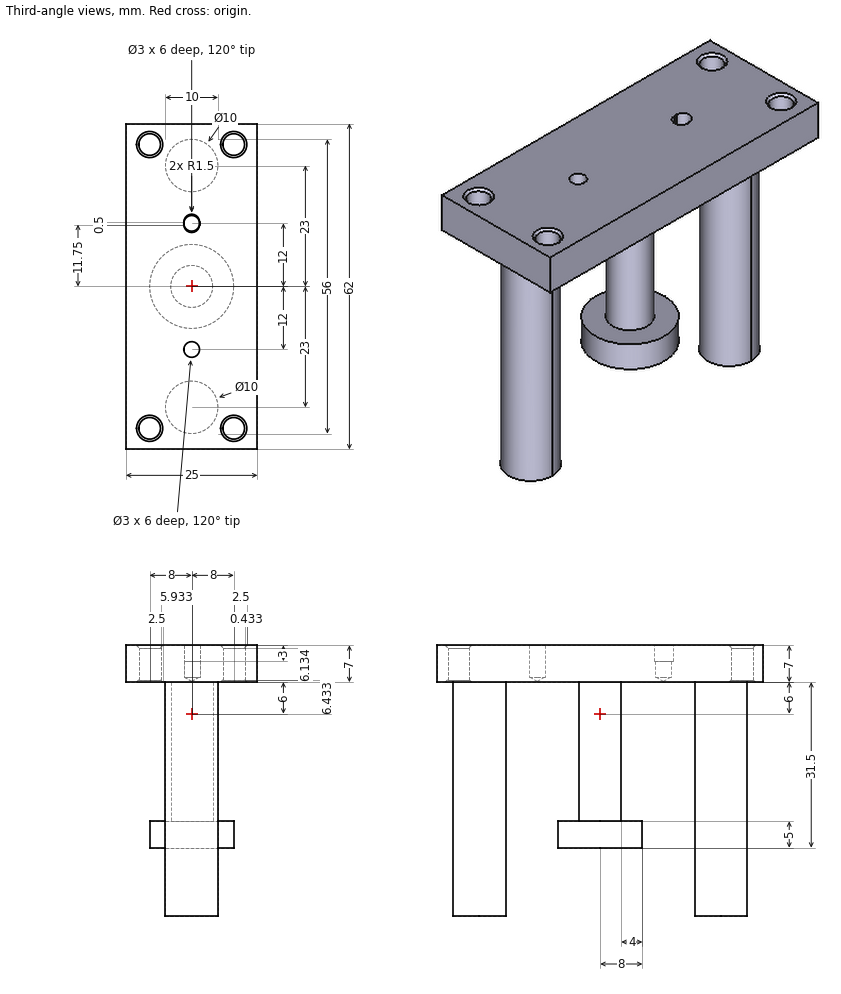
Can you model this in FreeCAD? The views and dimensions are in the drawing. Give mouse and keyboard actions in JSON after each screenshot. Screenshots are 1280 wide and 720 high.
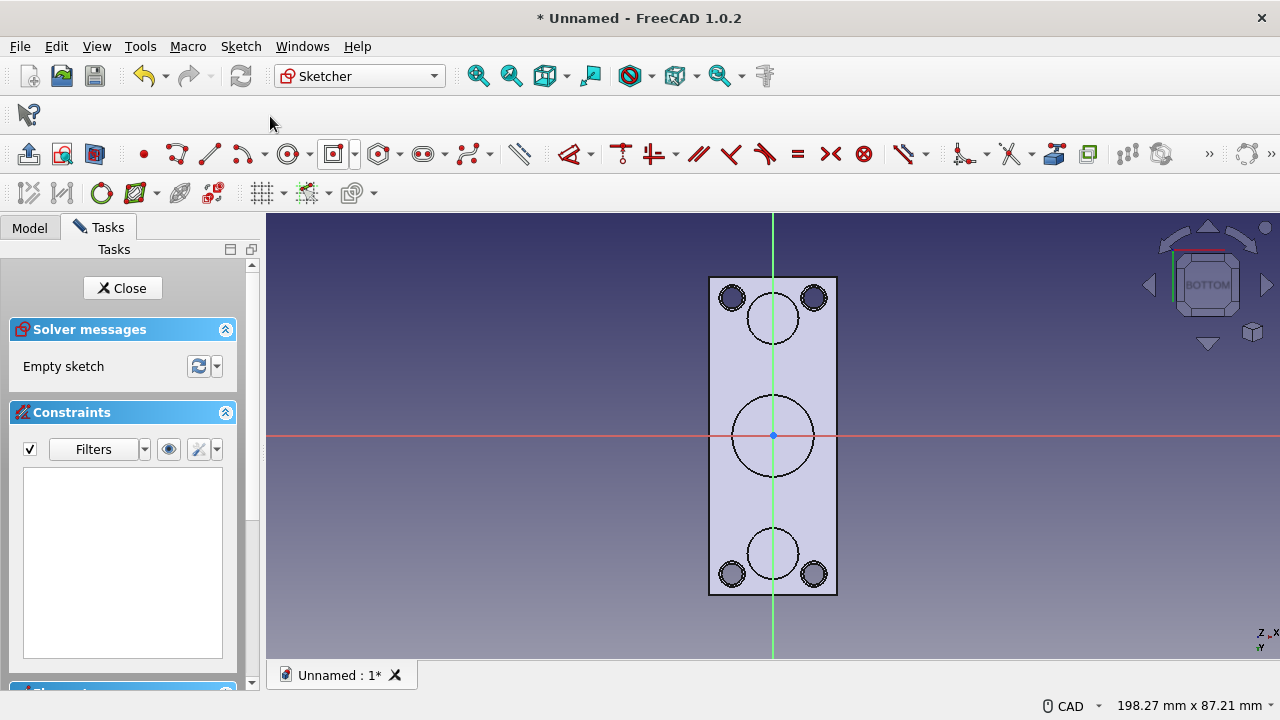
{"action": "left_click", "coordinate": [332, 154]}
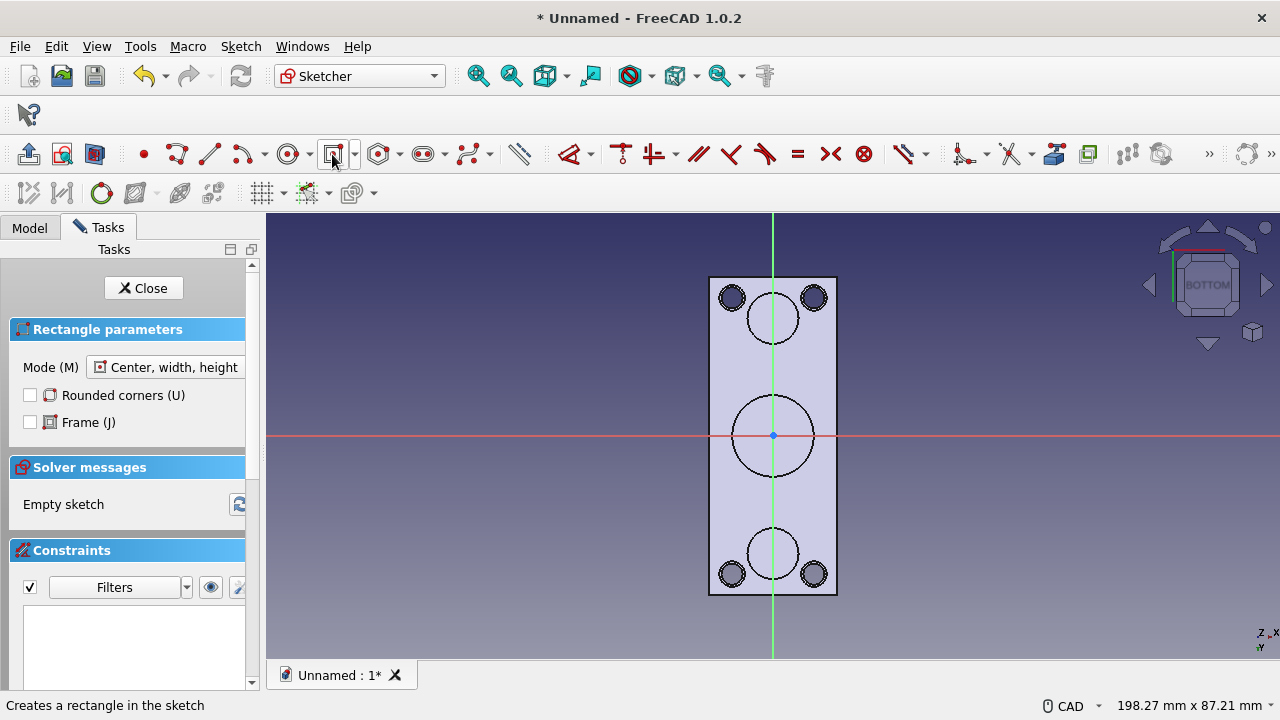
{"action": "left_click", "coordinate": [773, 436]}
{"action": "left_click", "coordinate": [799, 293]}
{"action": "key", "text": "Escape"}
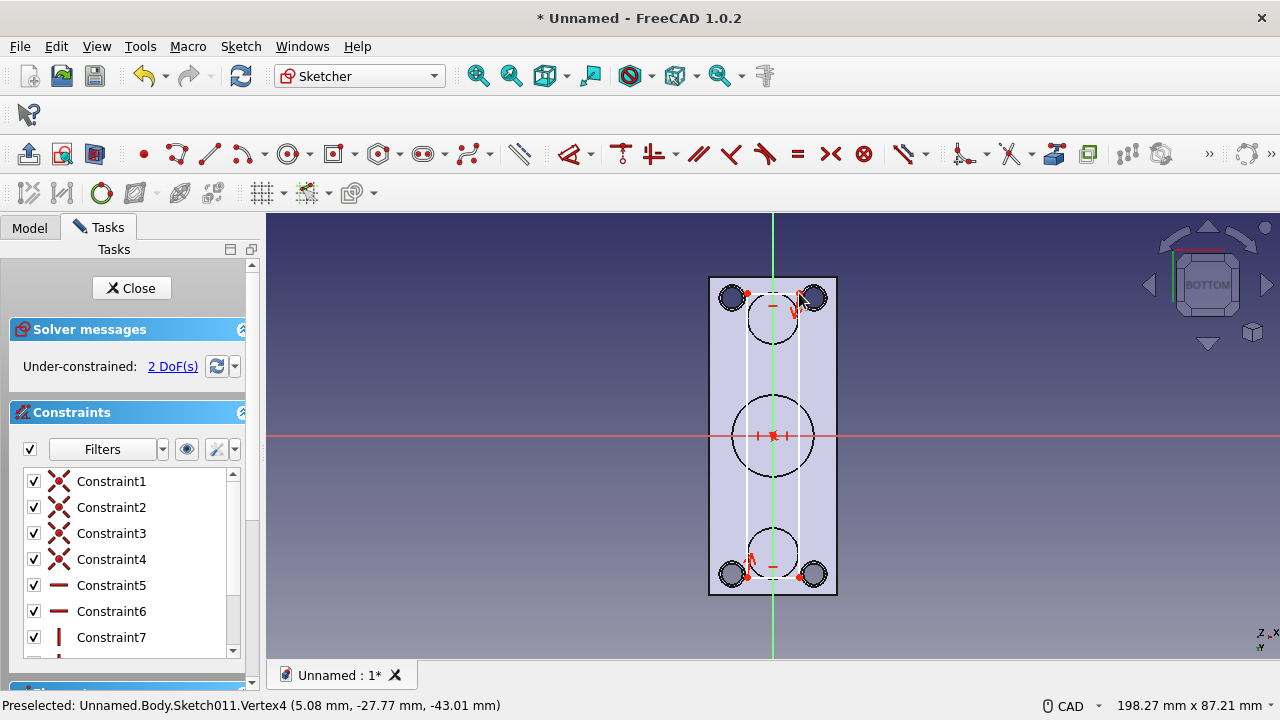
{"action": "left_click", "coordinate": [568, 154]}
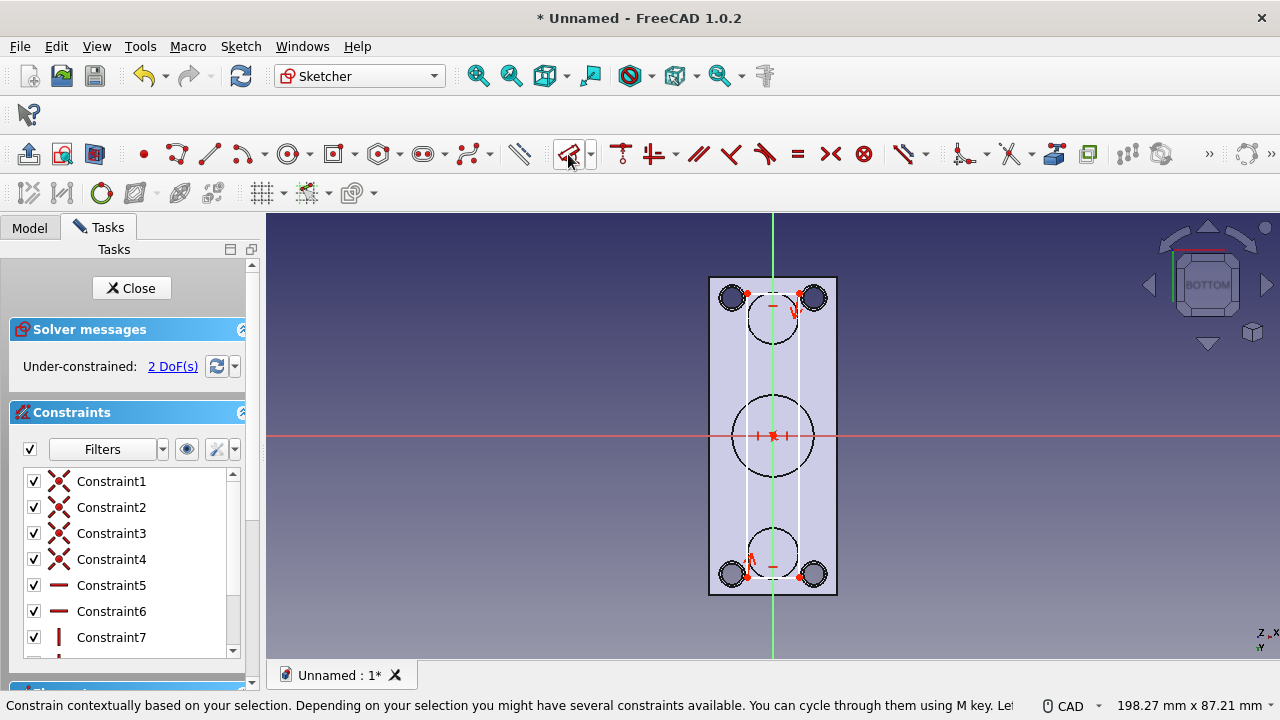
{"action": "scroll", "coordinate": [763, 578], "scroll_direction": "up", "scroll_amount": 2}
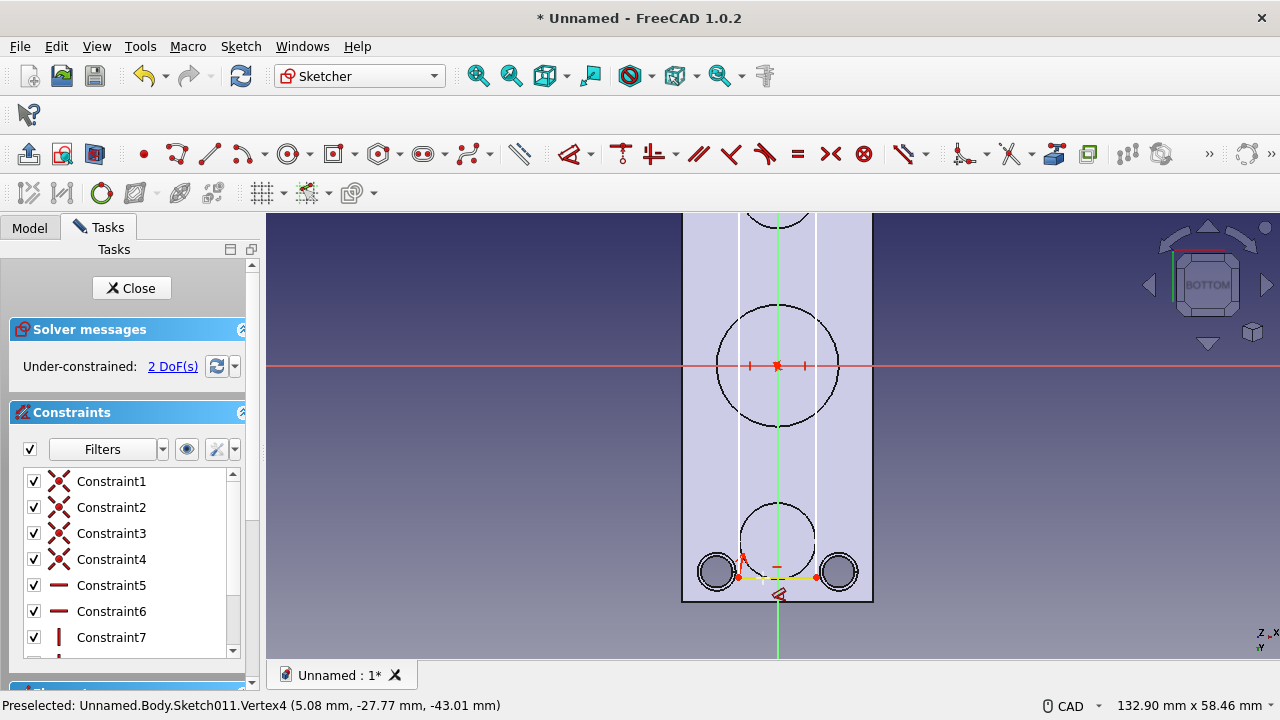
{"action": "left_click", "coordinate": [762, 578]}
{"action": "left_click", "coordinate": [760, 612]}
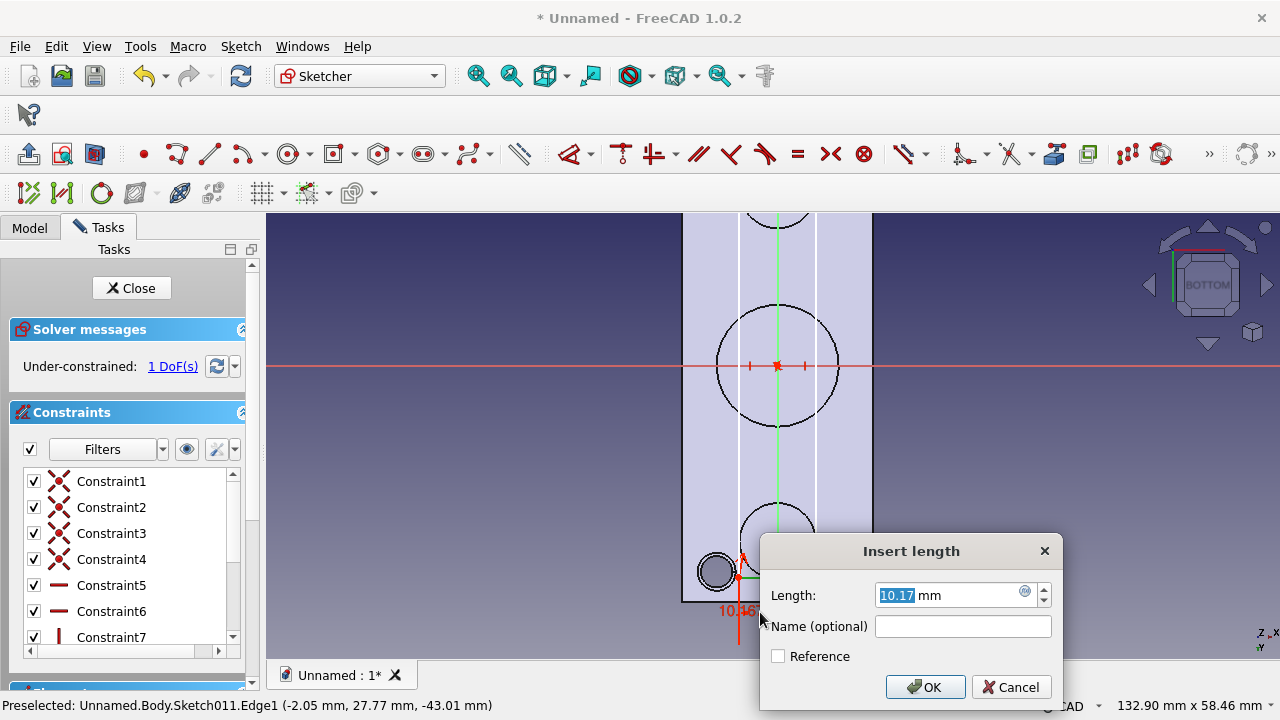
{"action": "type", "text": "10"}
{"action": "key", "text": "Return"}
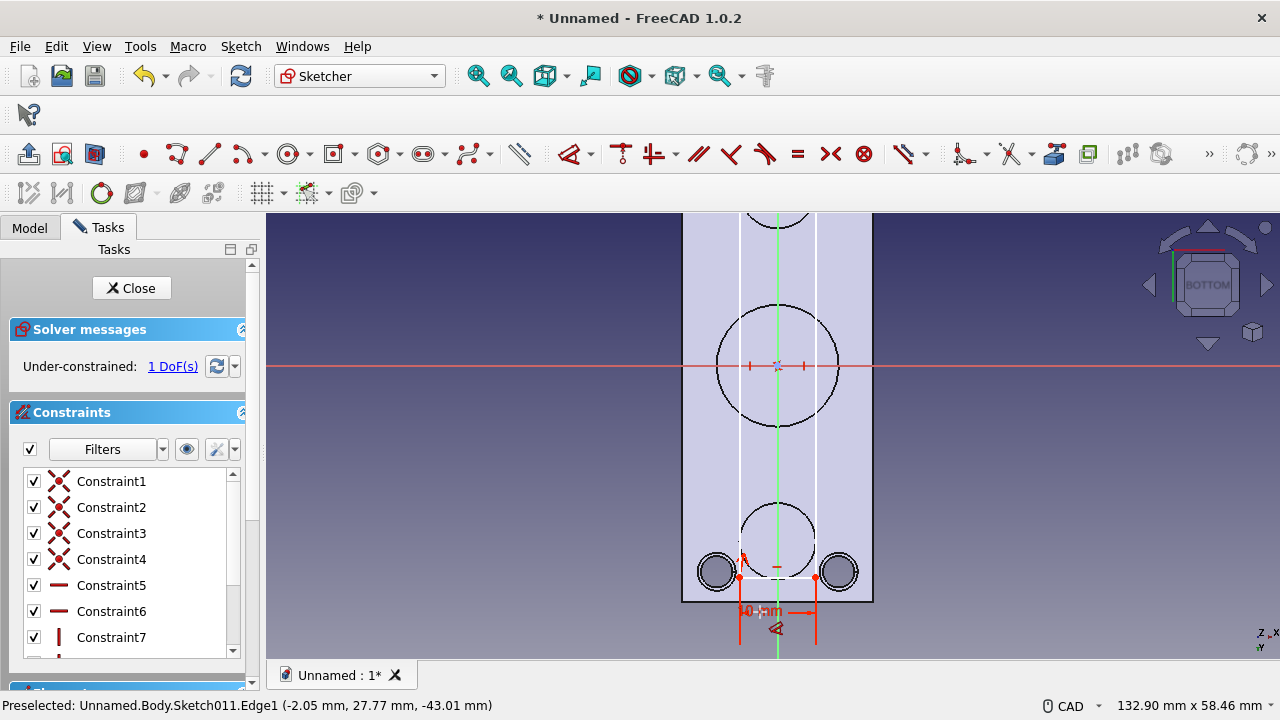
{"action": "left_click", "coordinate": [816, 450]}
{"action": "left_click", "coordinate": [850, 409]}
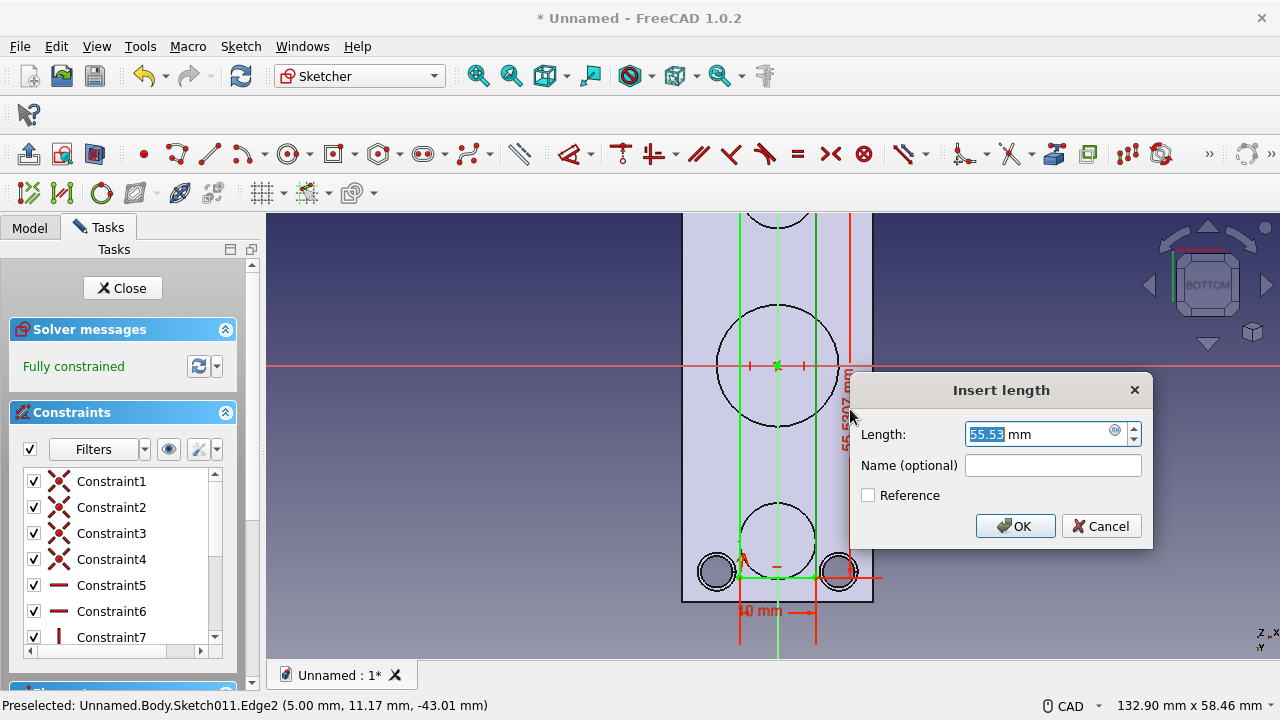
{"action": "type", "text": "56"}
{"action": "key", "text": "Return"}
{"action": "key", "text": "Escape"}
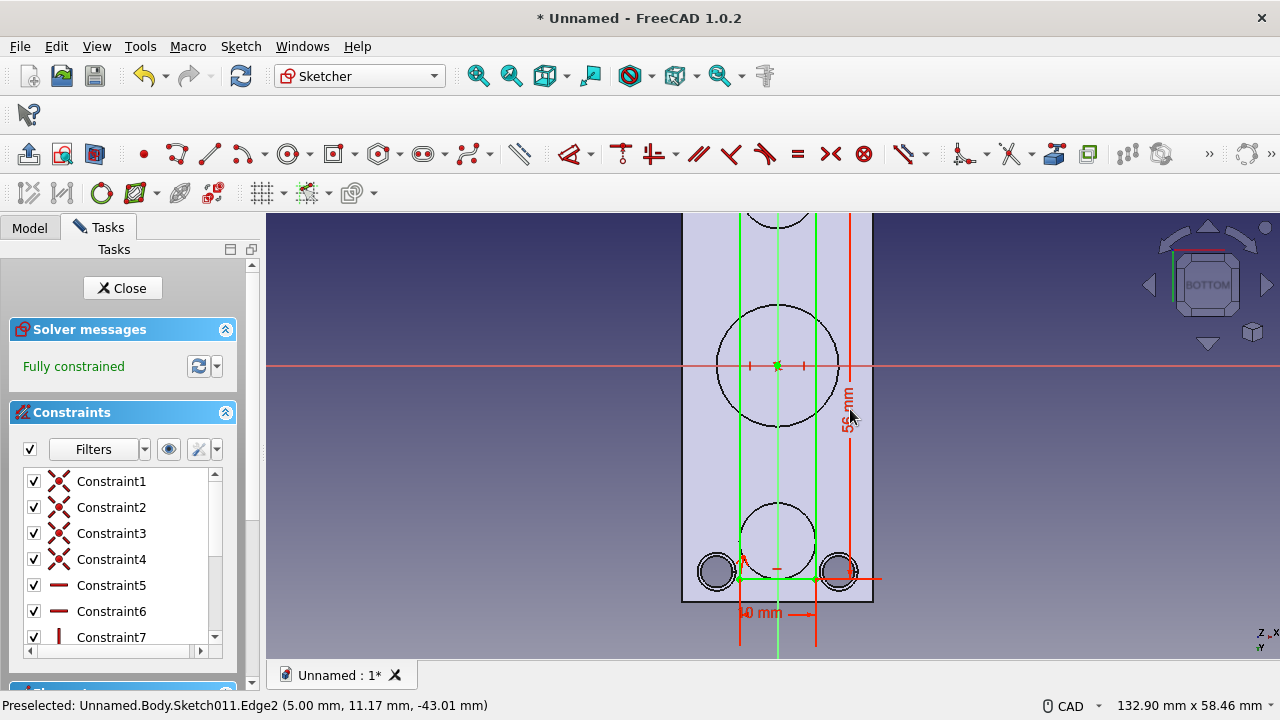
{"action": "left_click", "coordinate": [123, 288]}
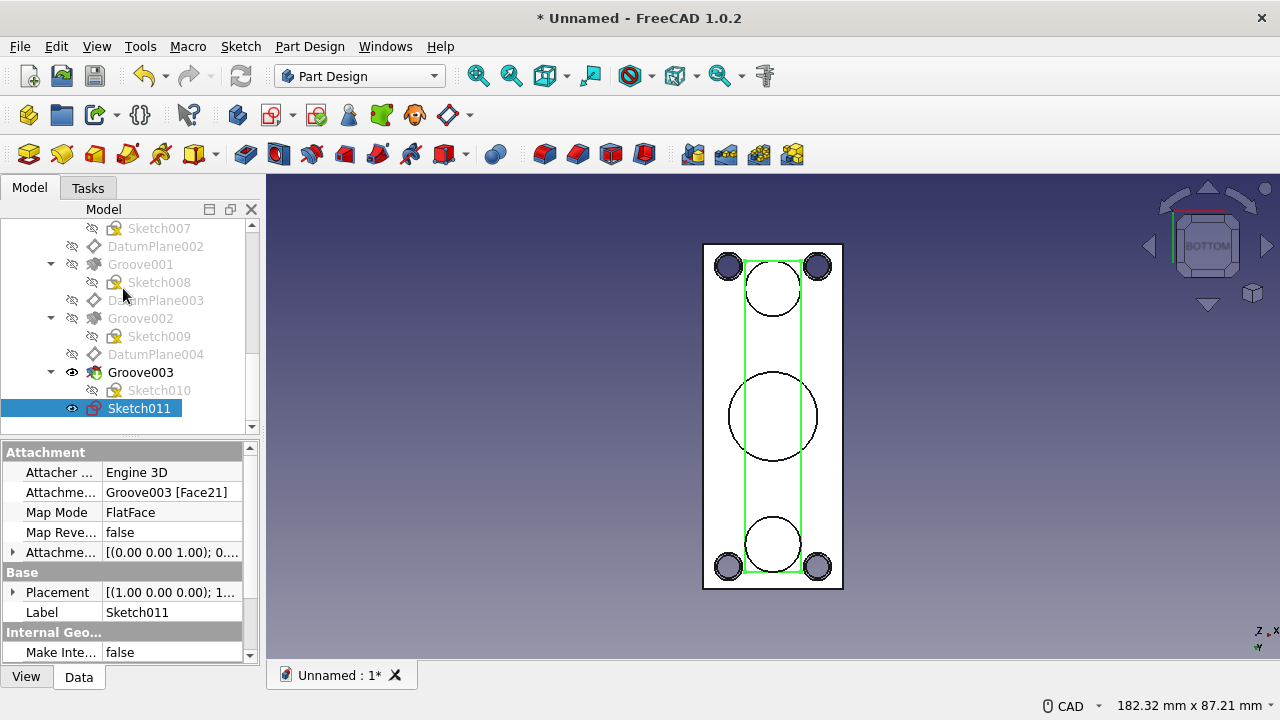
{"action": "left_click", "coordinate": [246, 154]}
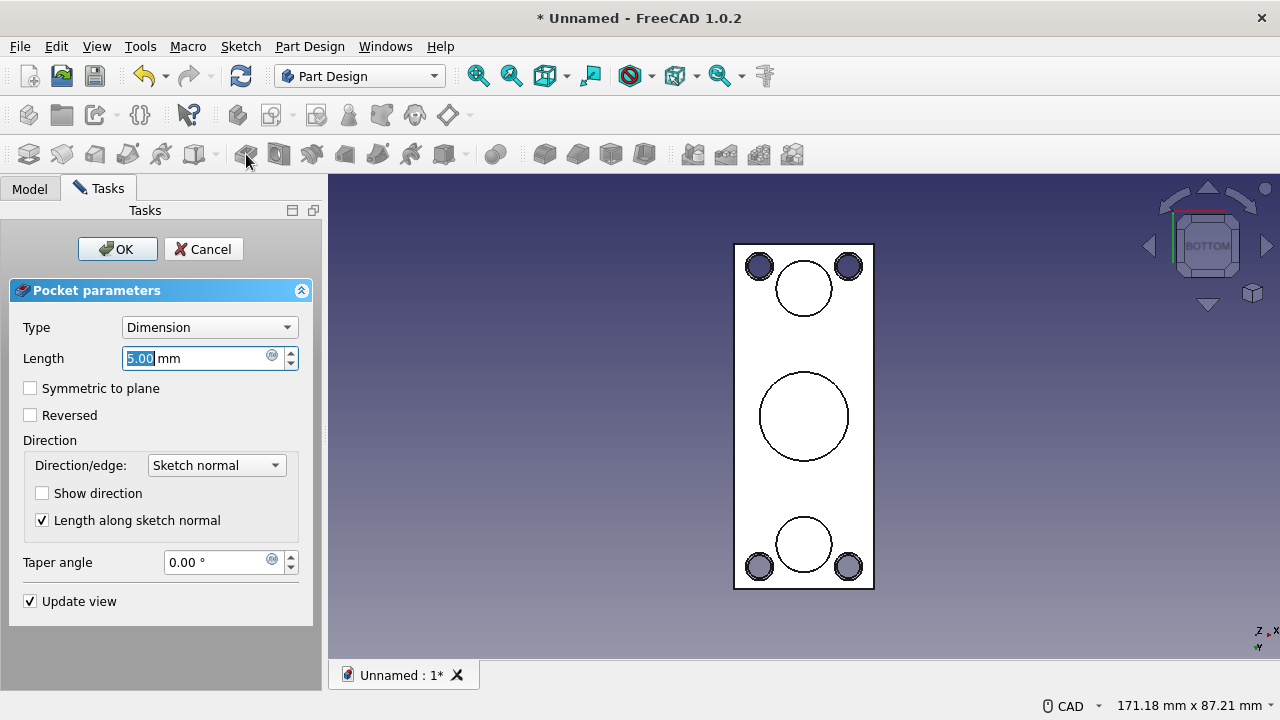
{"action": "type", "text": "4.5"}
{"action": "key", "text": "Tab"}